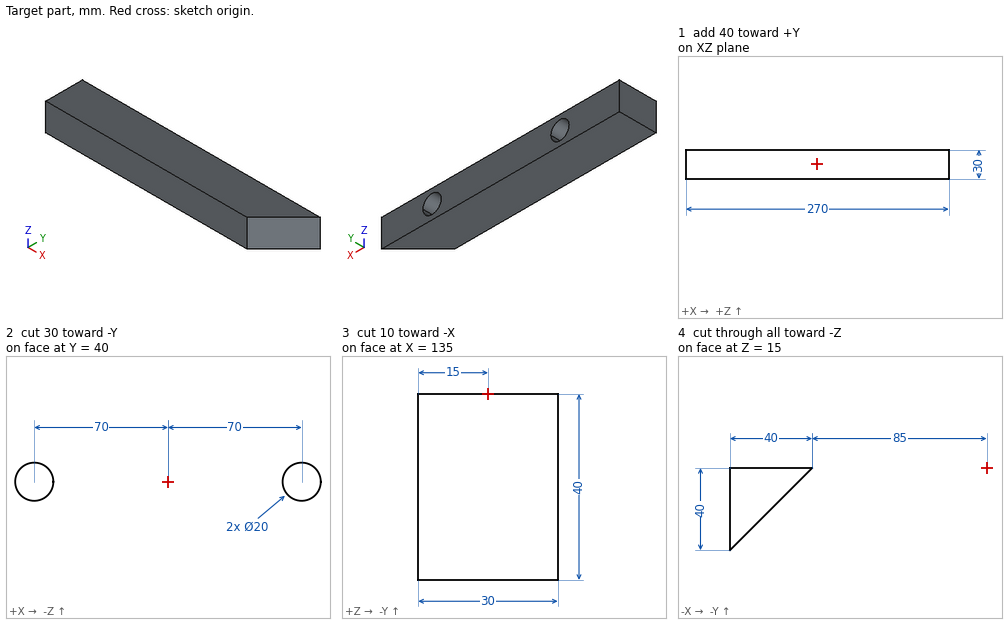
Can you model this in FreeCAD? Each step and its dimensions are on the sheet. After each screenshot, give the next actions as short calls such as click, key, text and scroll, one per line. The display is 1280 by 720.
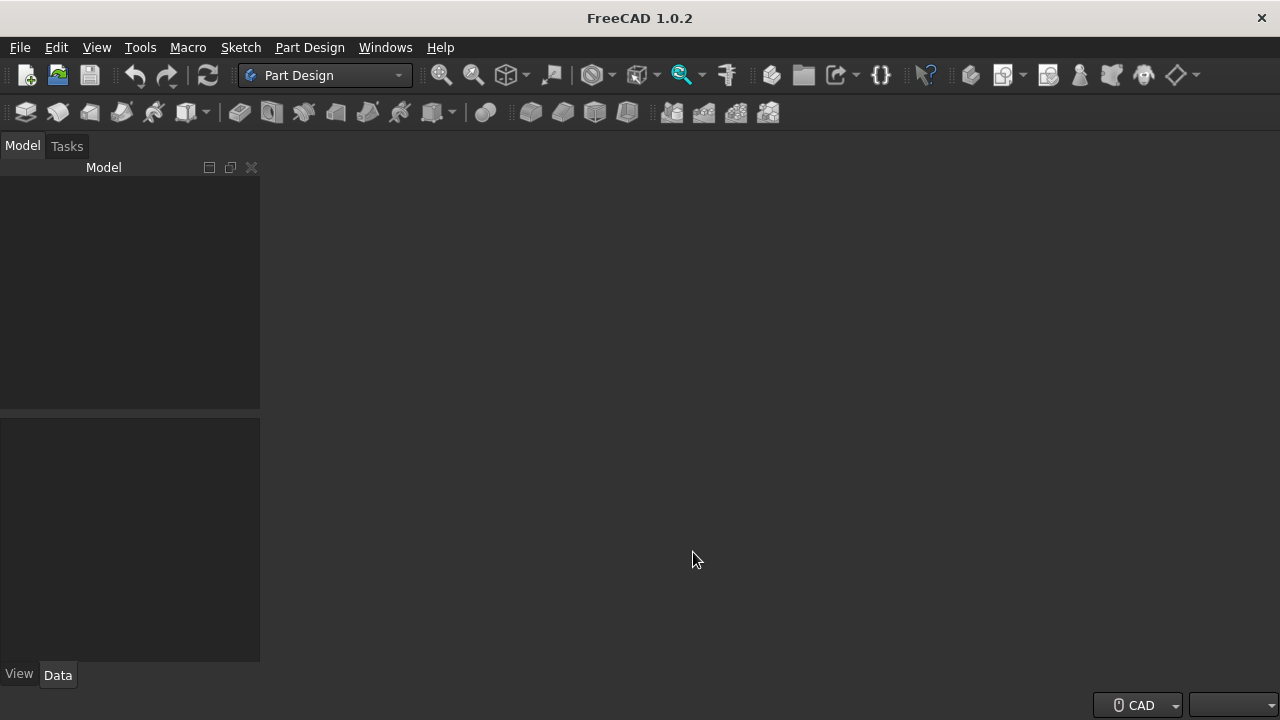
click(26, 76)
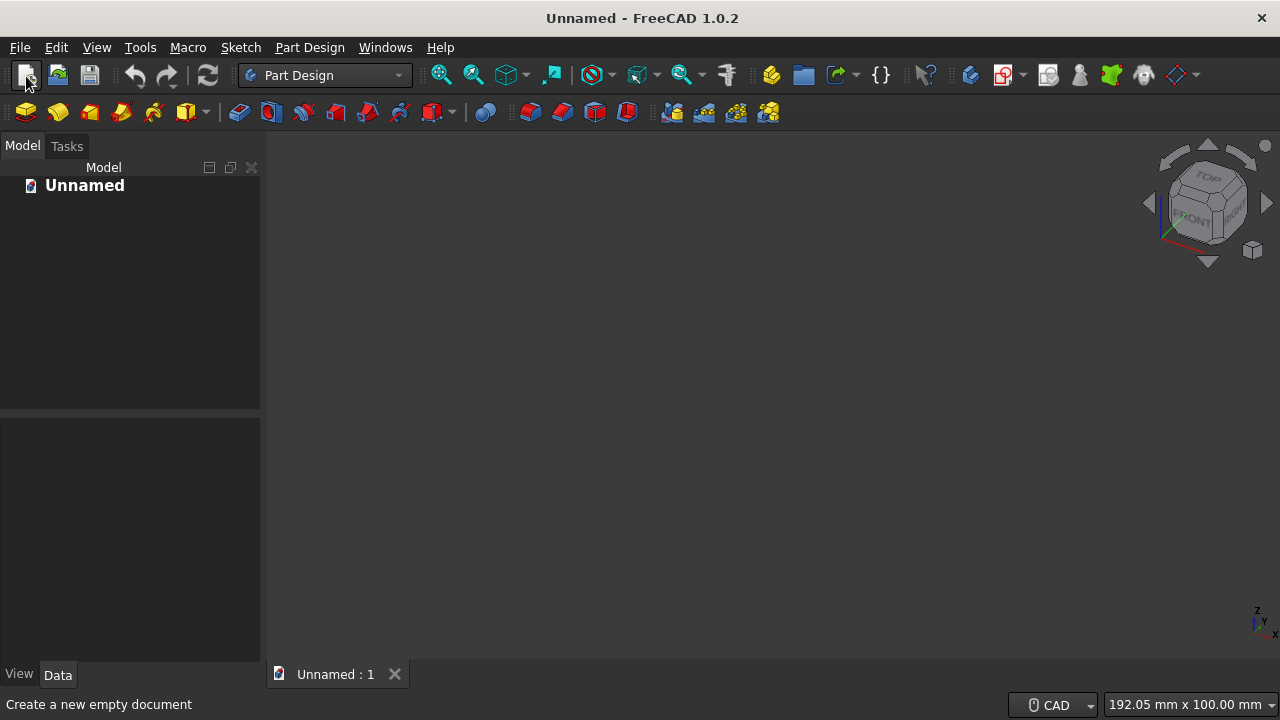
click(1004, 76)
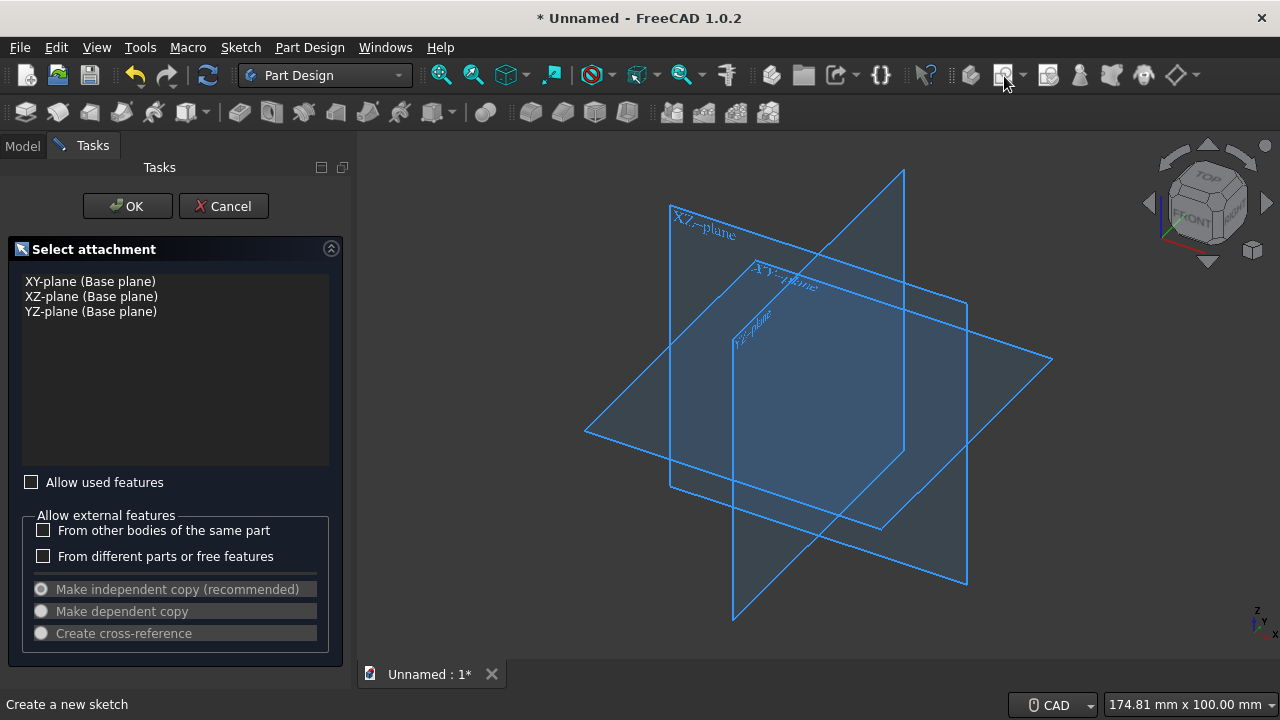
click(82, 296)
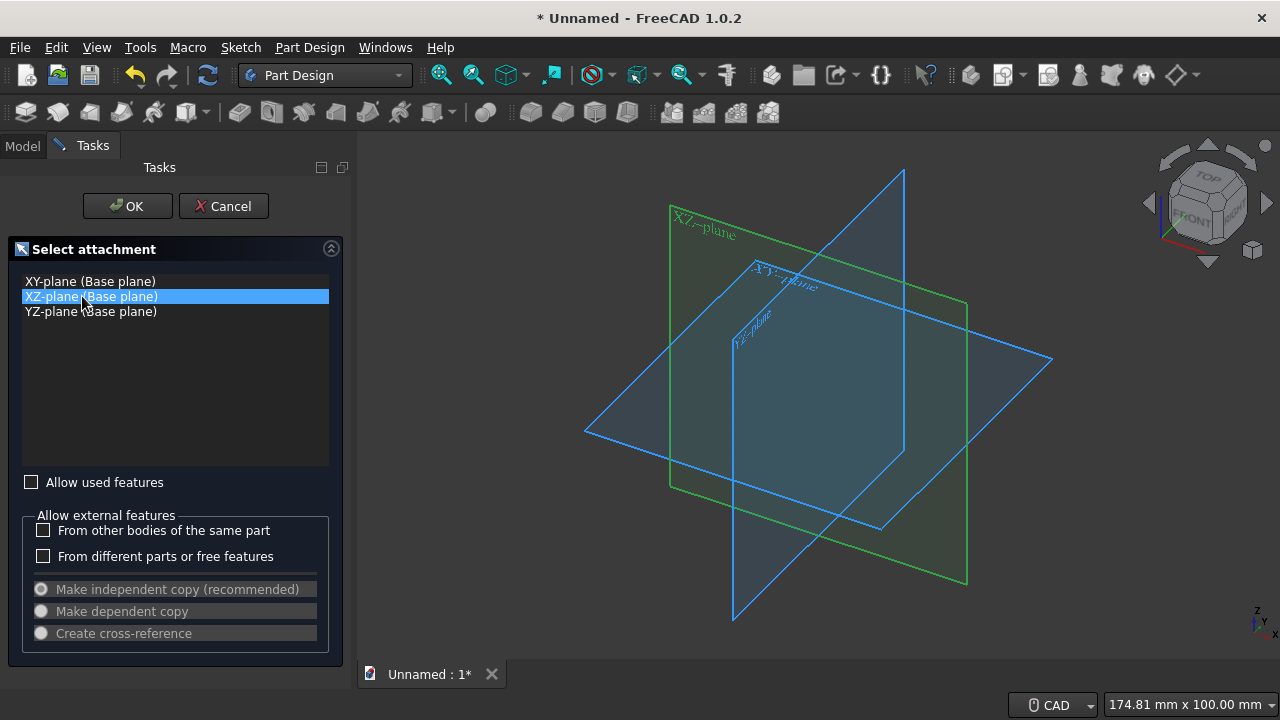
click(128, 206)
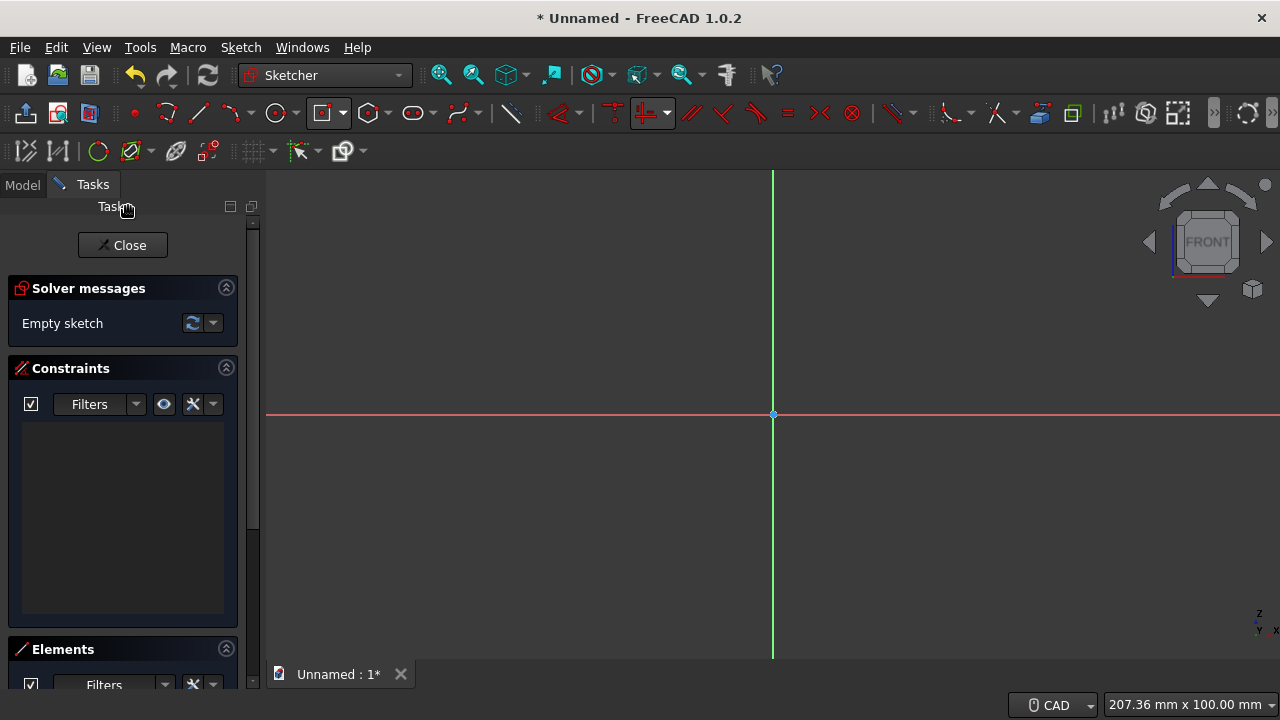
scroll(649, 414, down, 4)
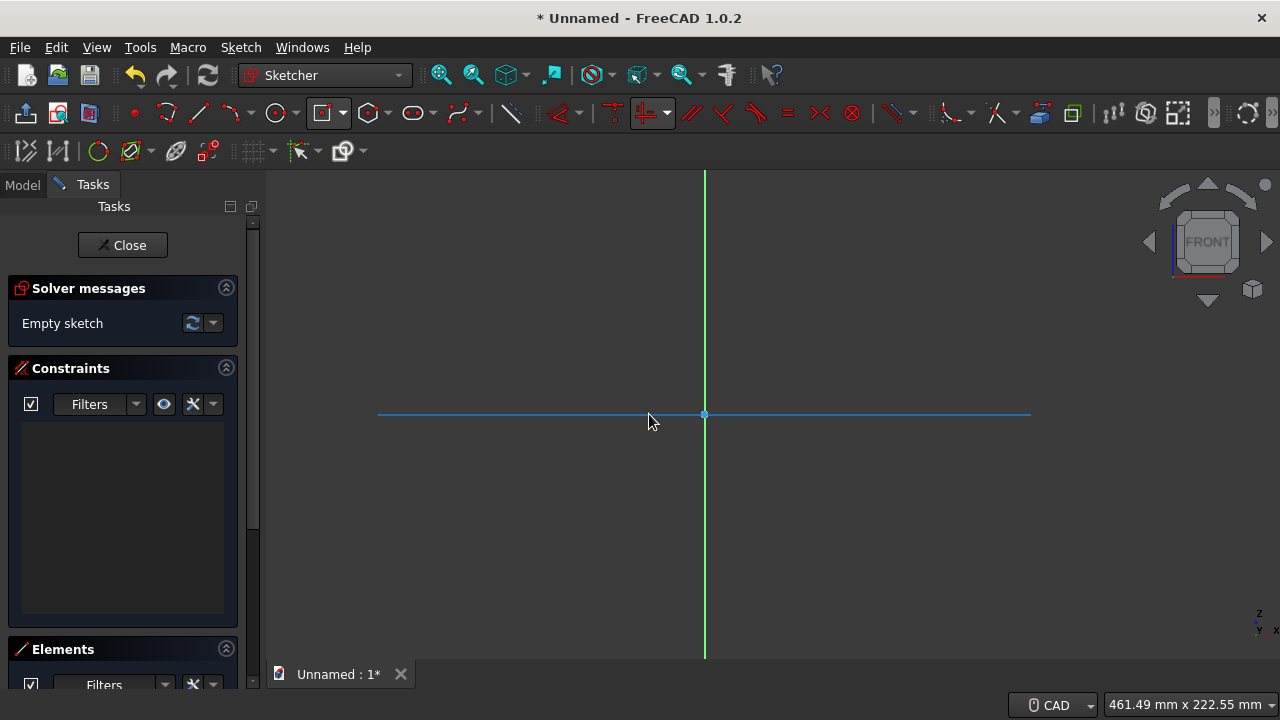
click(322, 114)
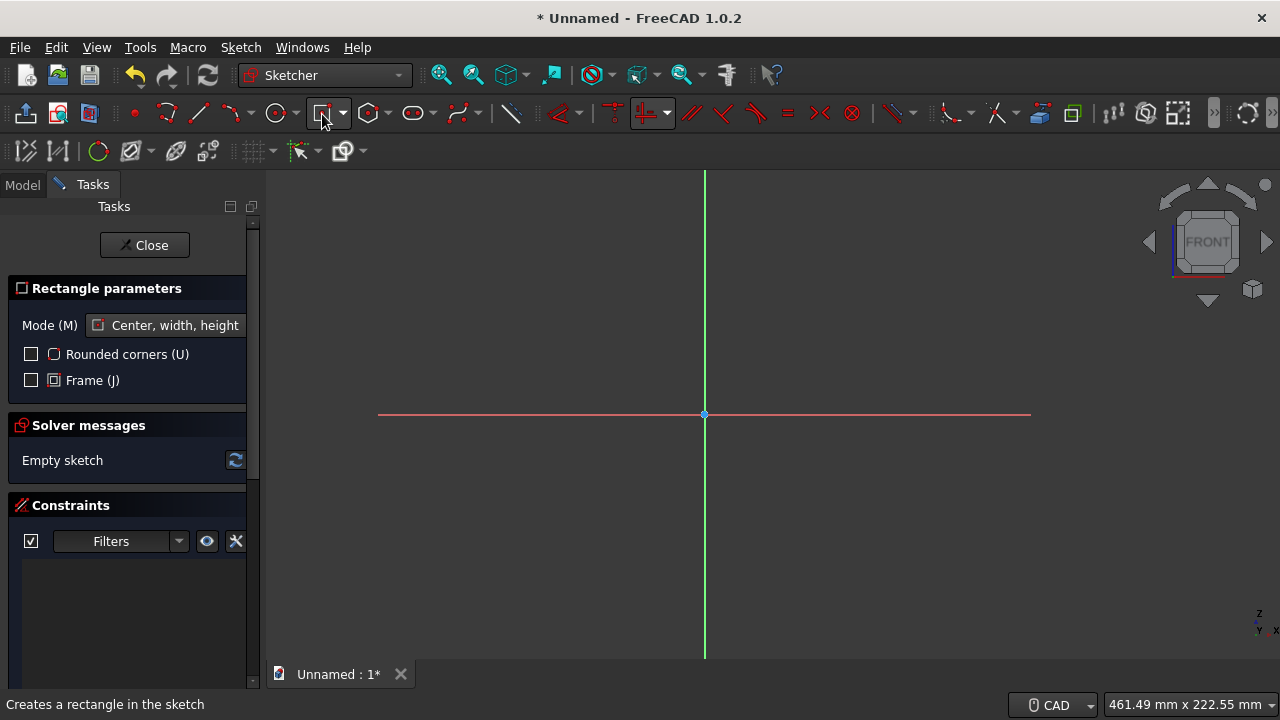
click(705, 414)
move(1002, 382)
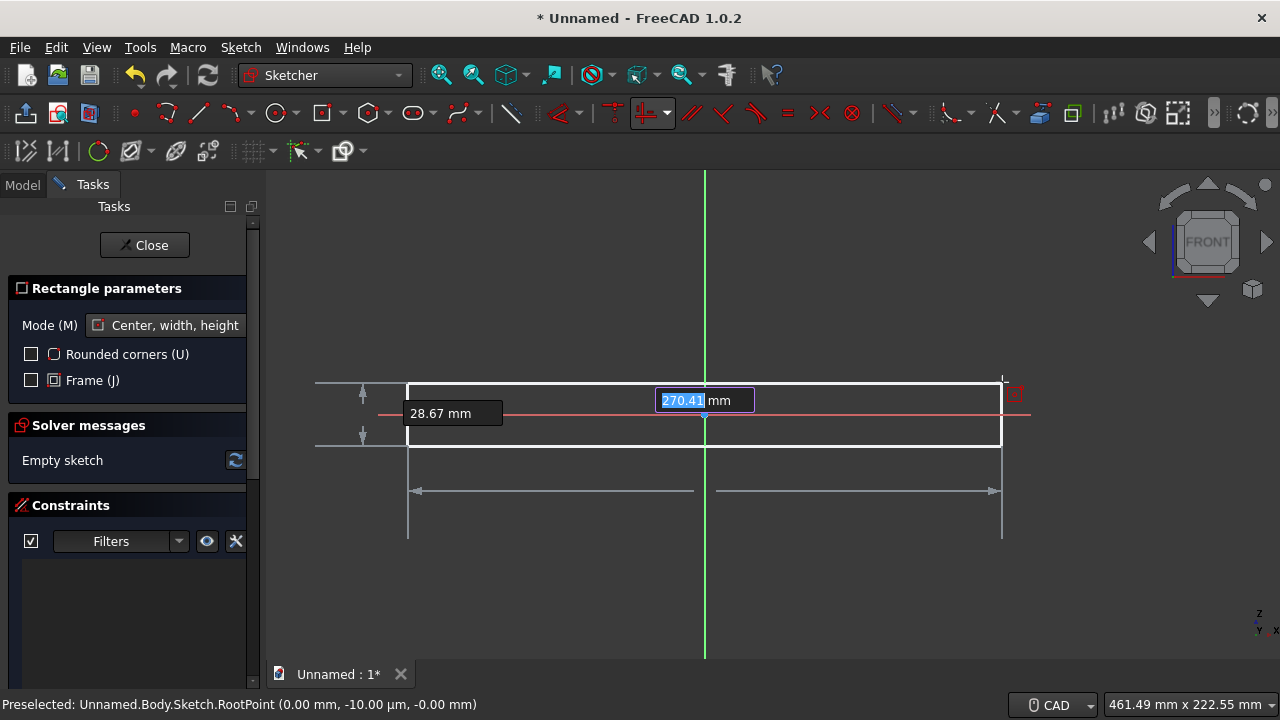
text(270)
key(Tab)
text(30)
key(Return)
key(Escape)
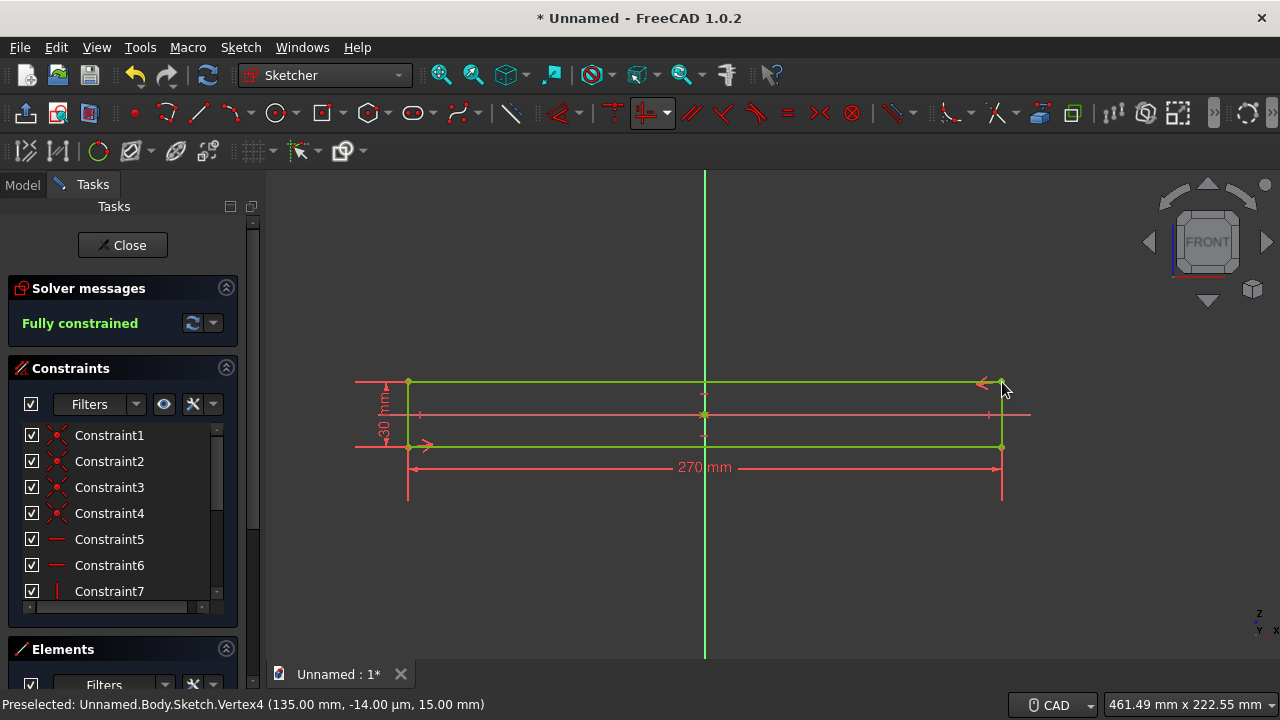
click(123, 245)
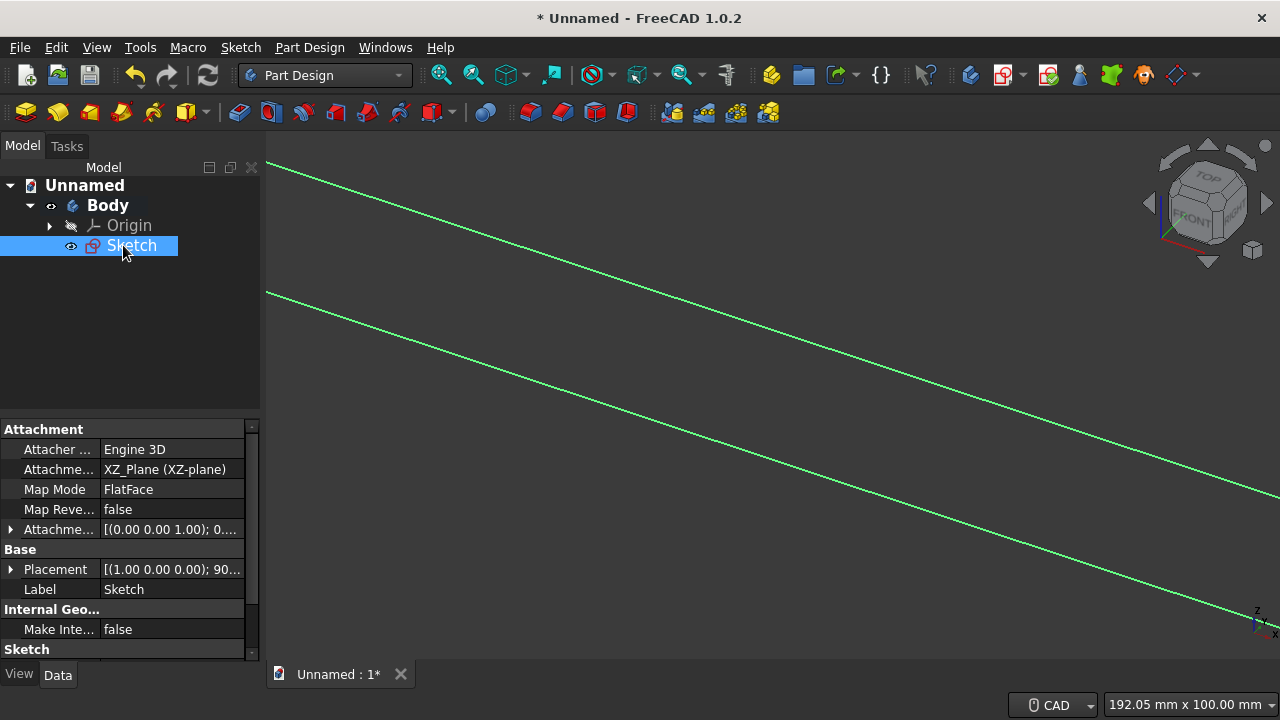
click(26, 112)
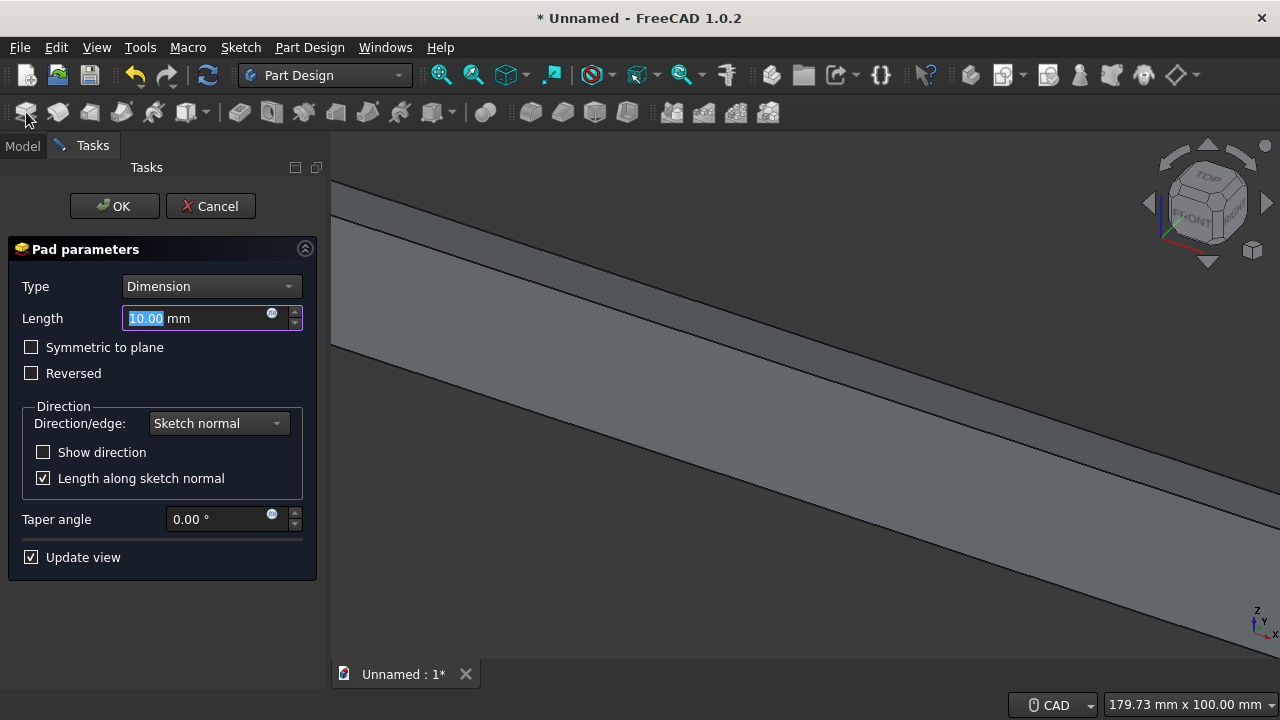
text(40)
key(Tab)